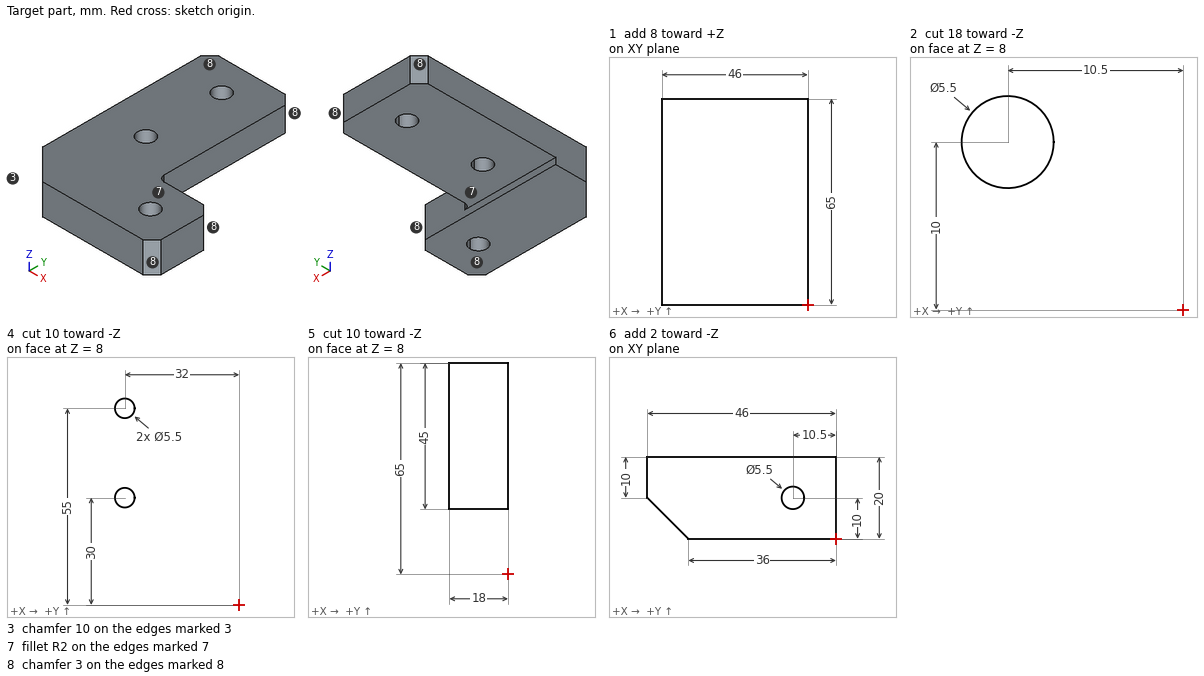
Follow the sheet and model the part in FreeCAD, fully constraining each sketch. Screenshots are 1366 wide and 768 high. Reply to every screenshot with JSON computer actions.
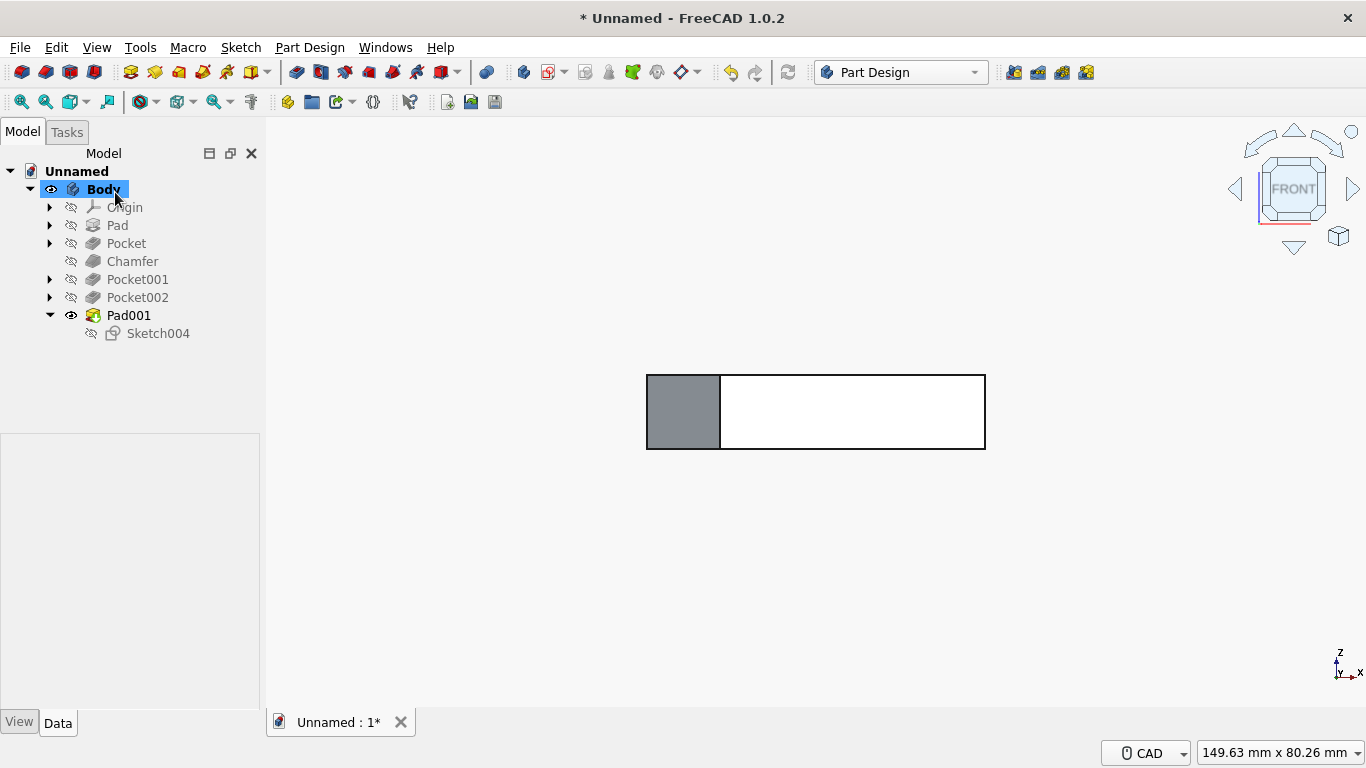
{"action": "key", "text": "3"}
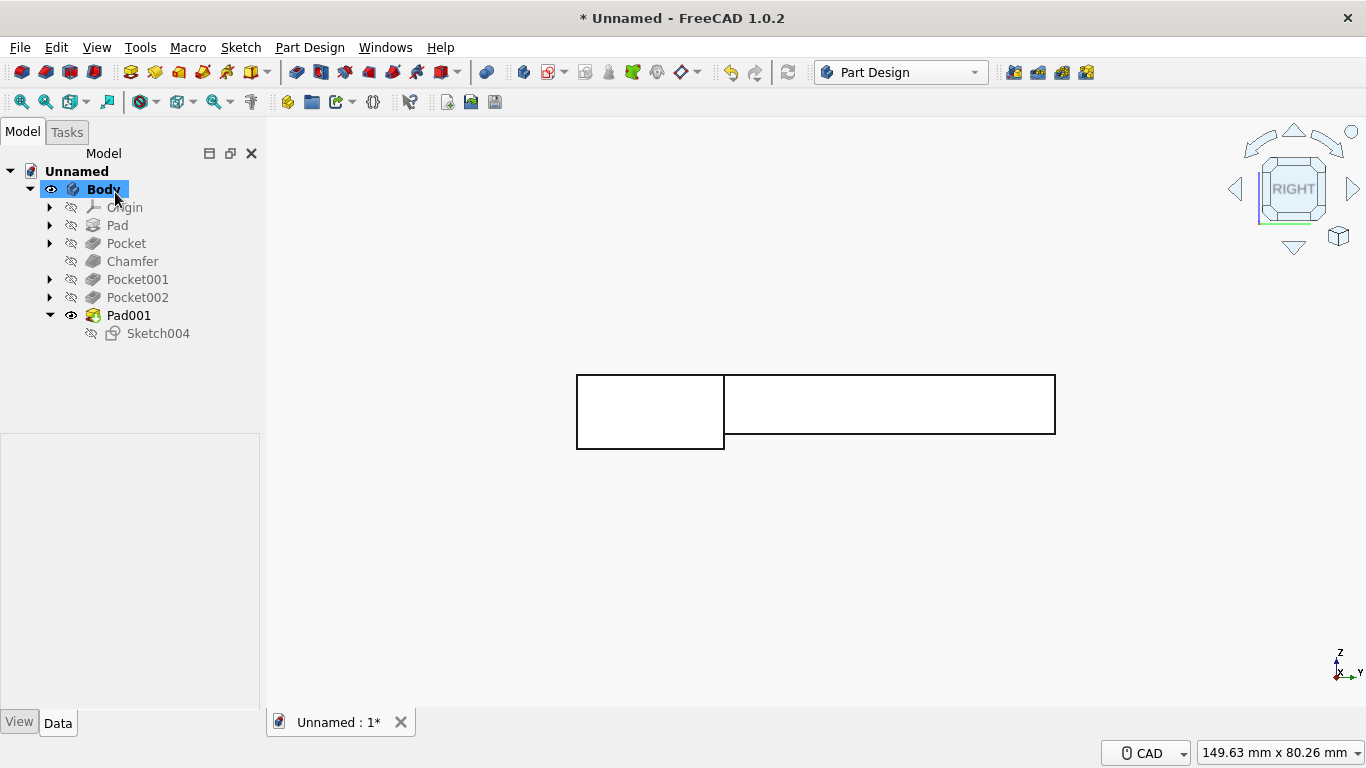
{"action": "left_click", "coordinate": [22, 102]}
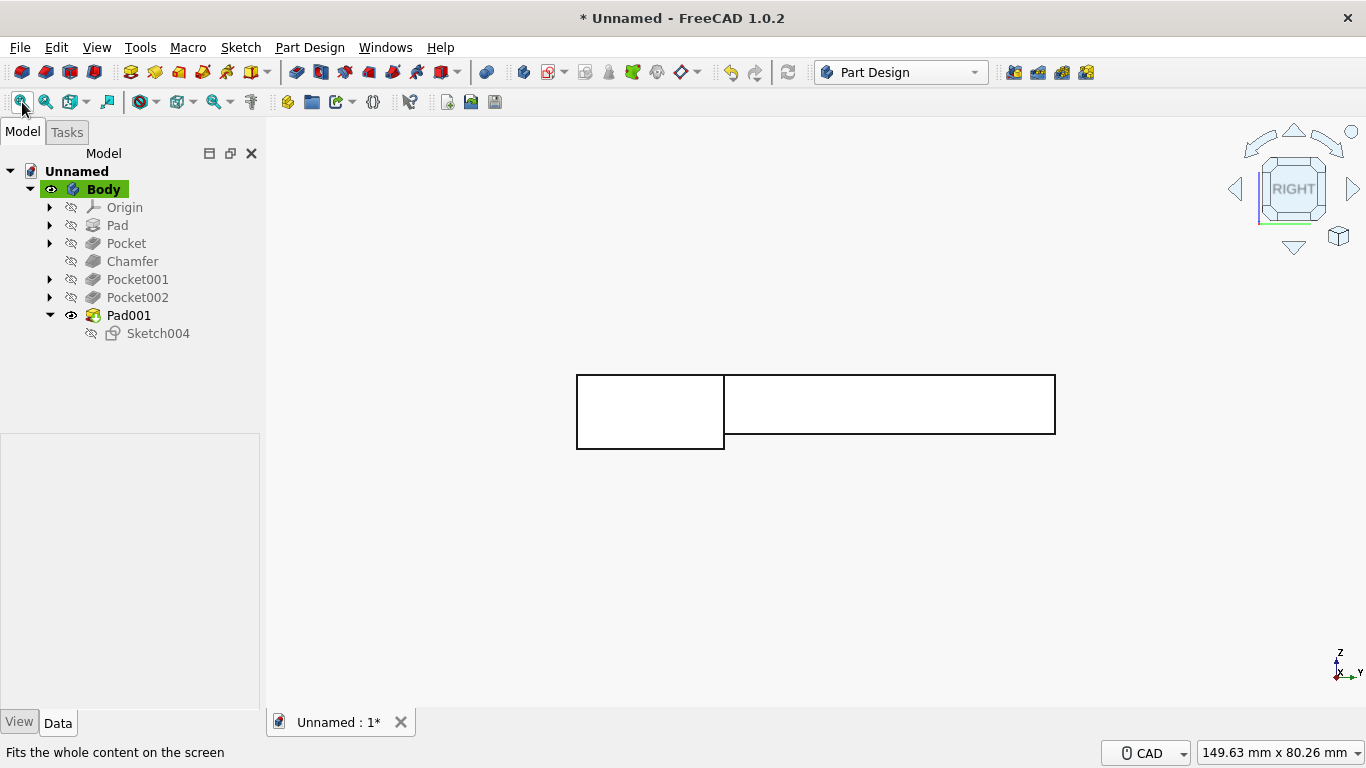
{"action": "key", "text": "5"}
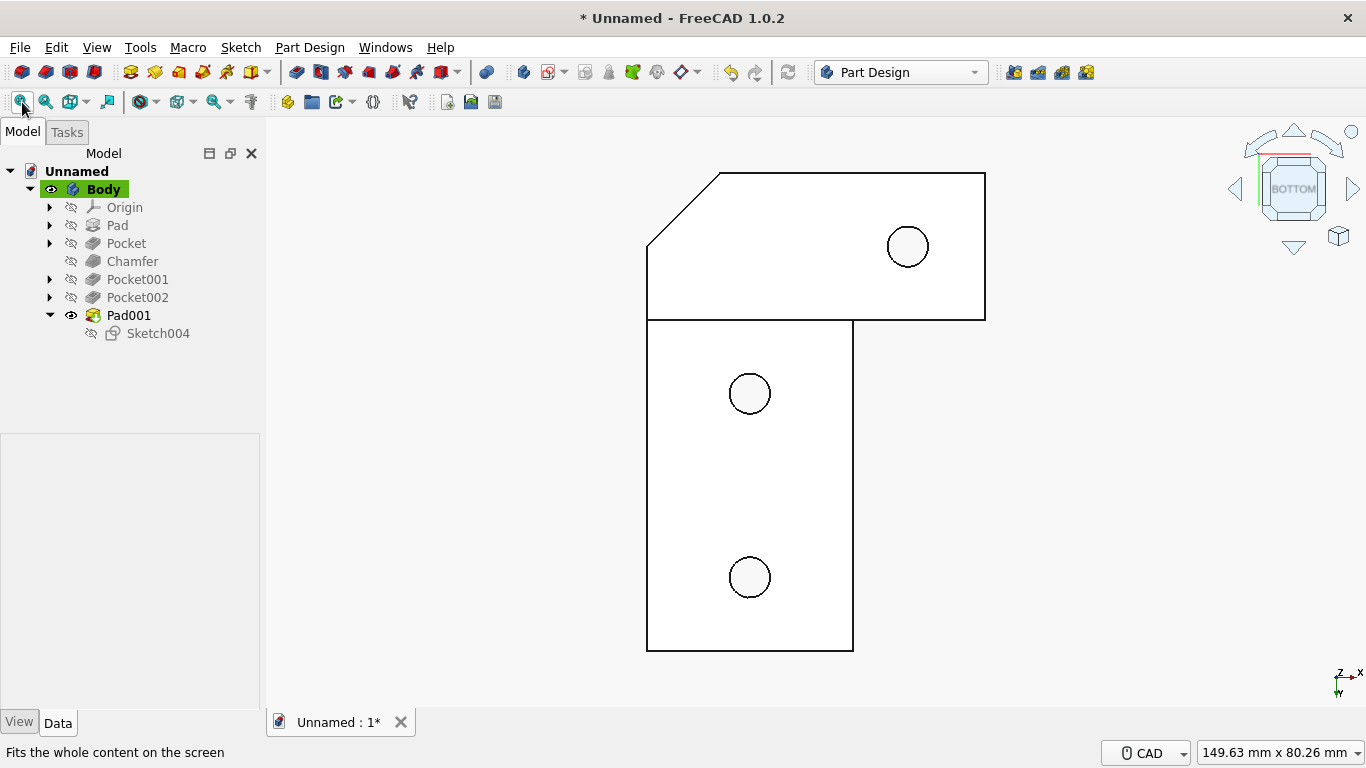
{"action": "key", "text": "4"}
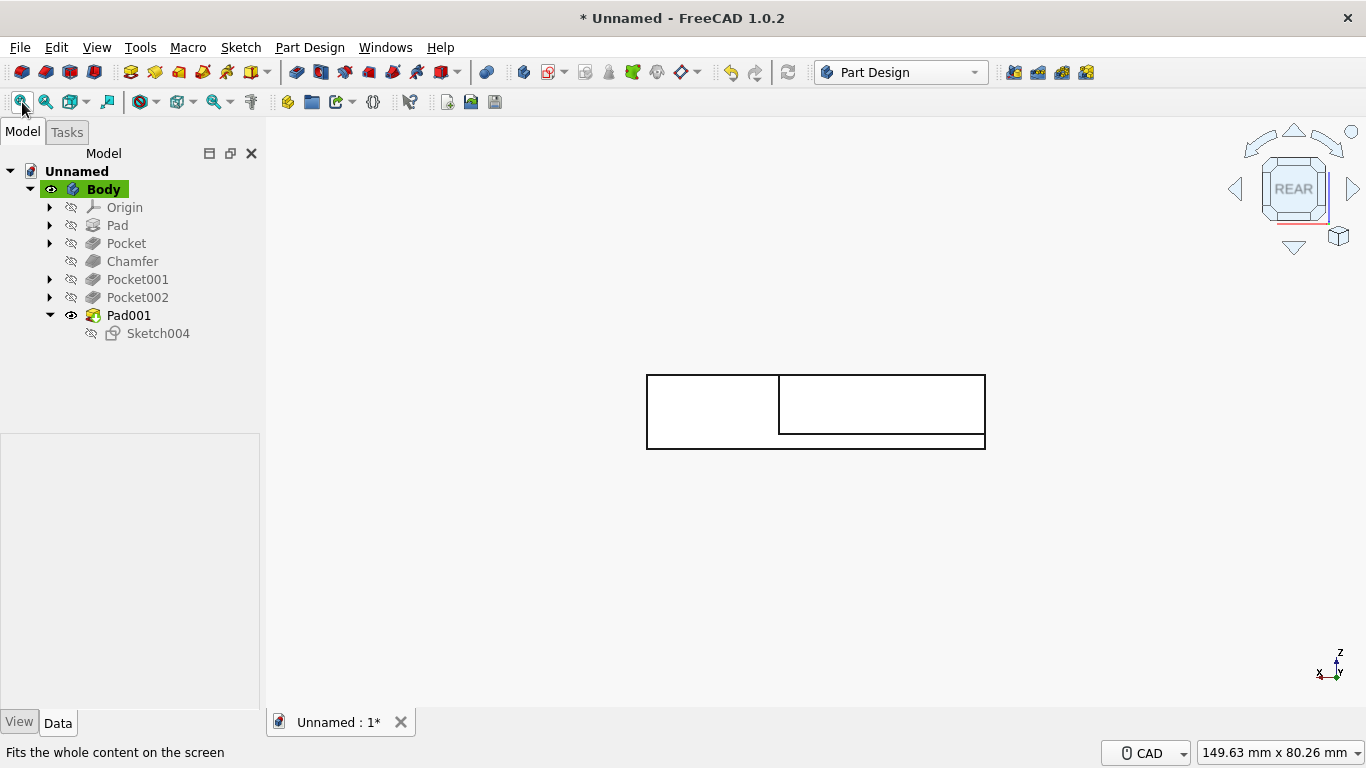
{"action": "left_click", "coordinate": [22, 102]}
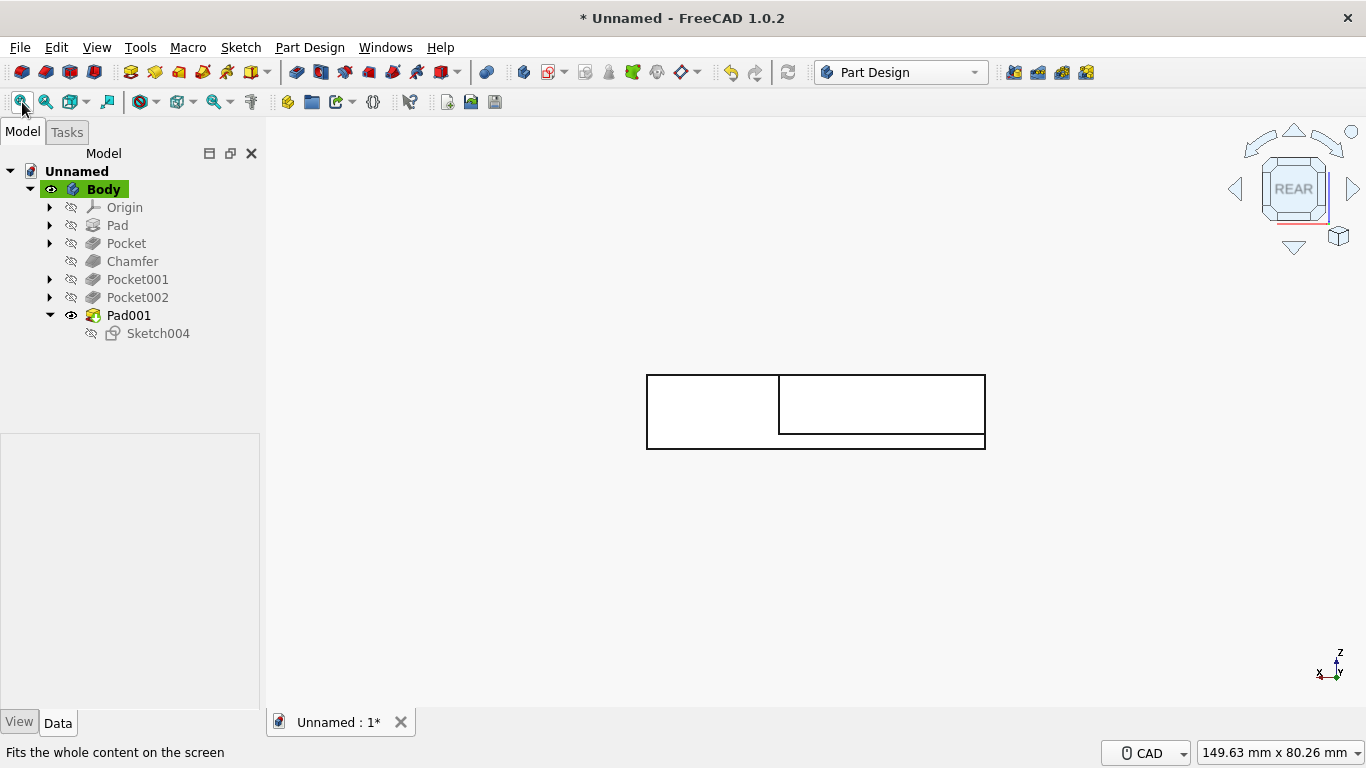
{"action": "key", "text": "6"}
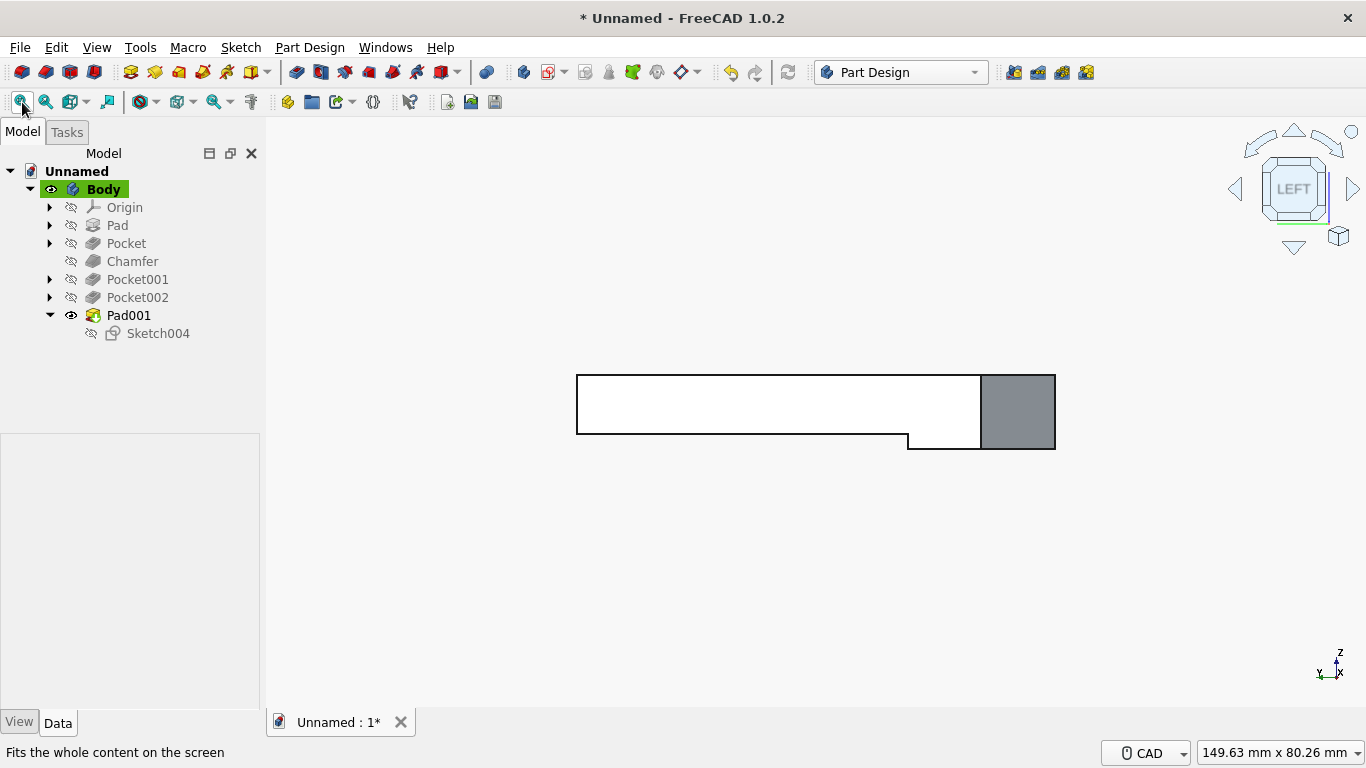
{"action": "left_click", "coordinate": [22, 102]}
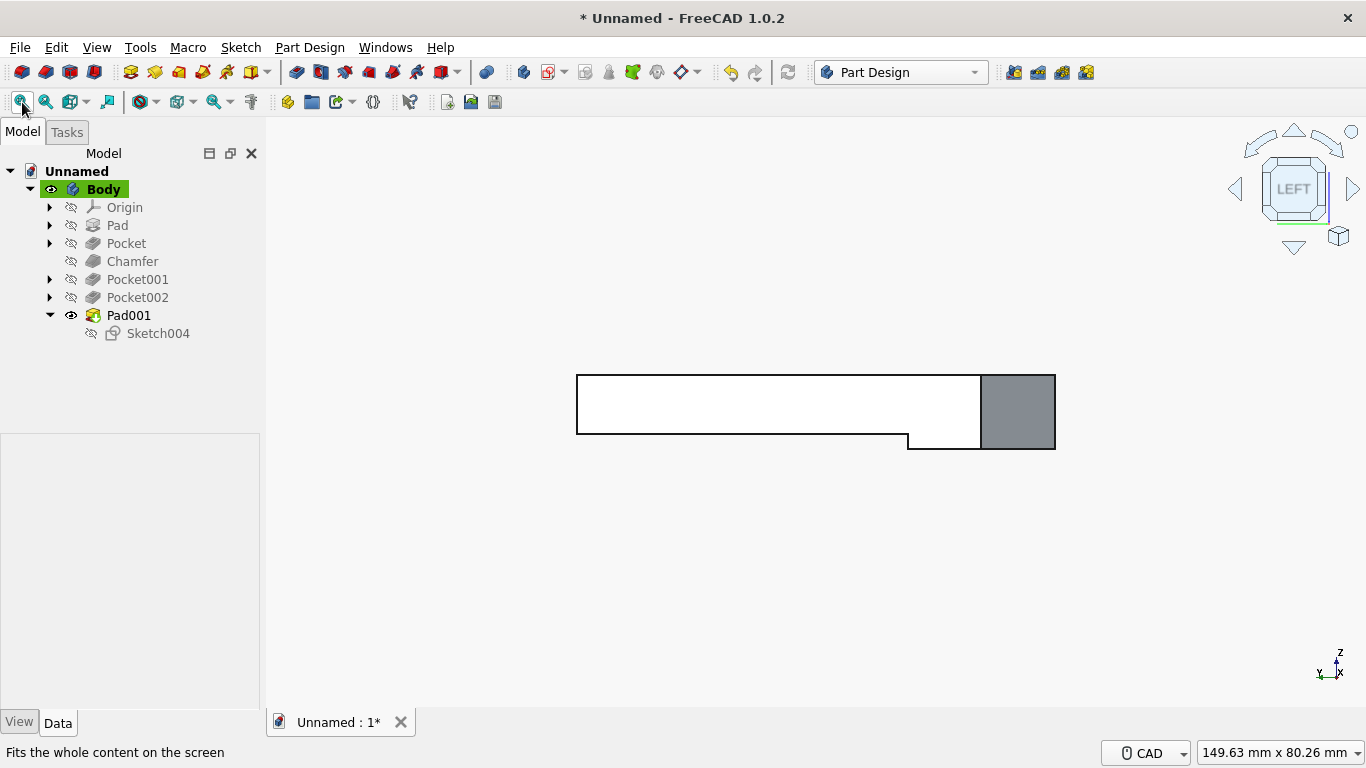
{"action": "key", "text": "v 3"}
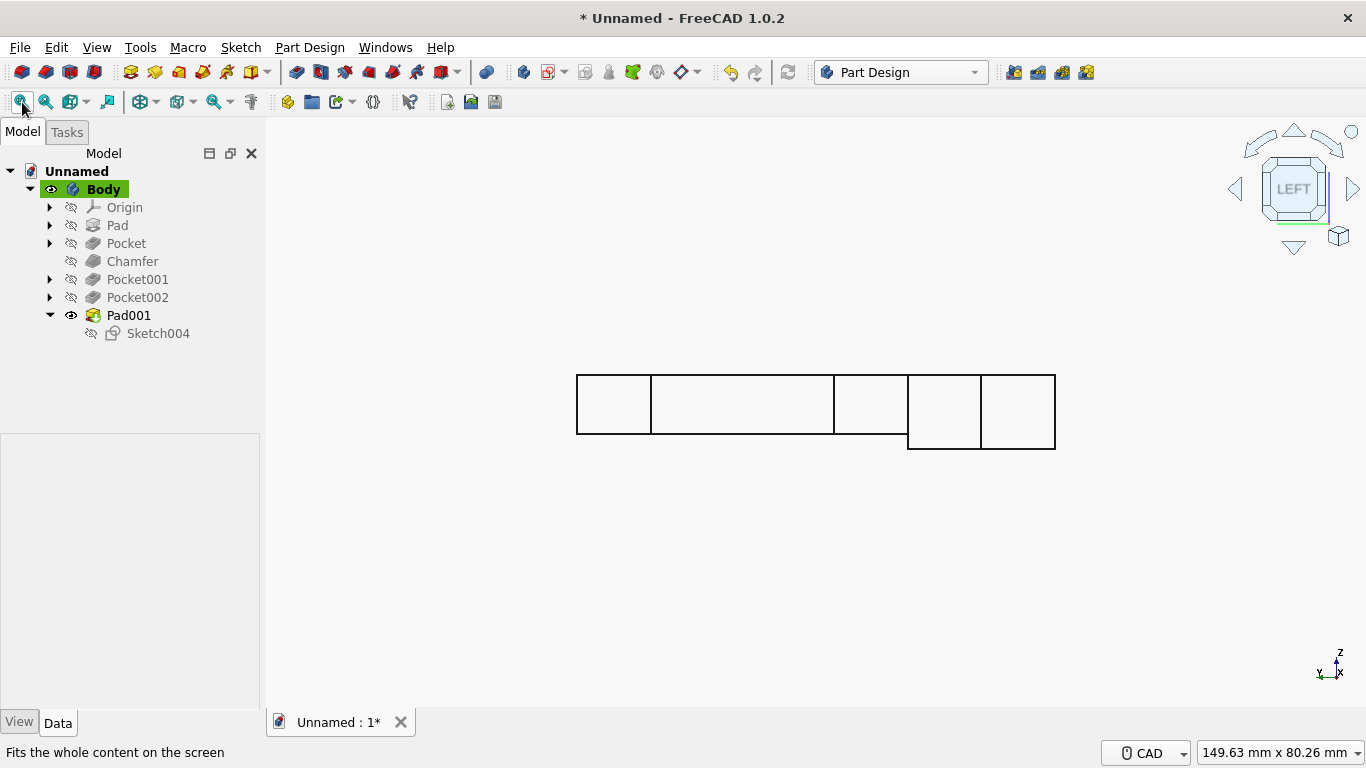
{"action": "key", "text": "0"}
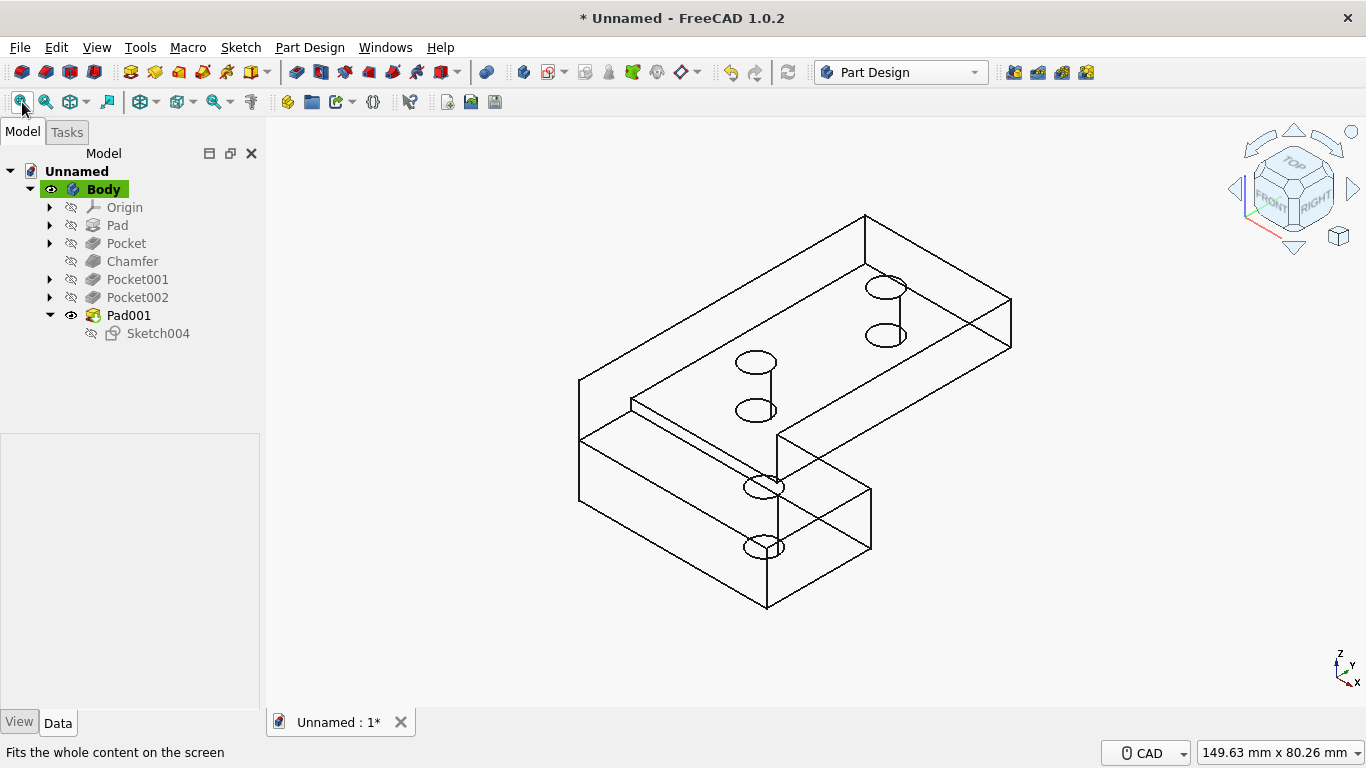
{"action": "left_click", "coordinate": [777, 458]}